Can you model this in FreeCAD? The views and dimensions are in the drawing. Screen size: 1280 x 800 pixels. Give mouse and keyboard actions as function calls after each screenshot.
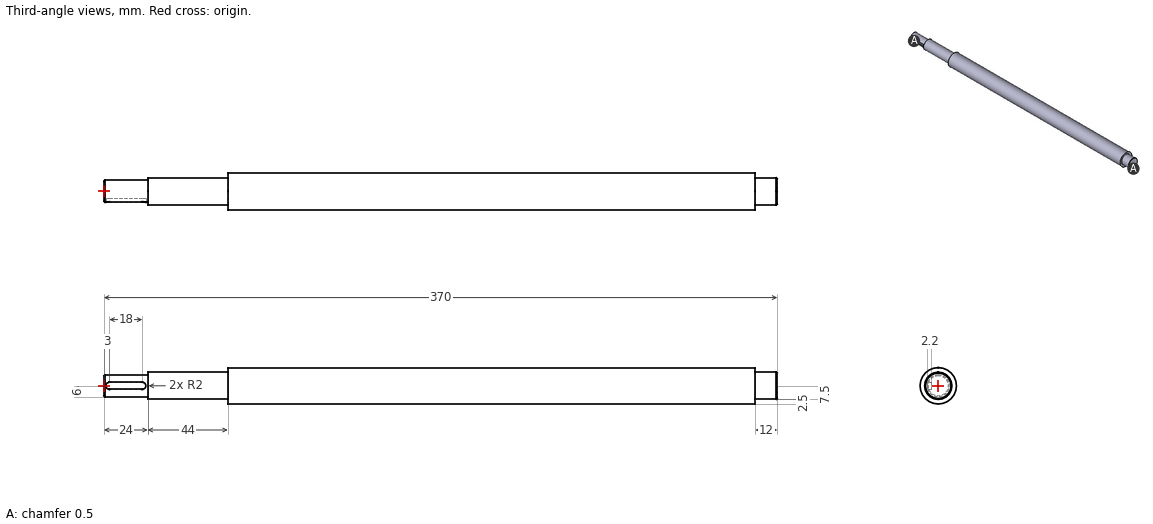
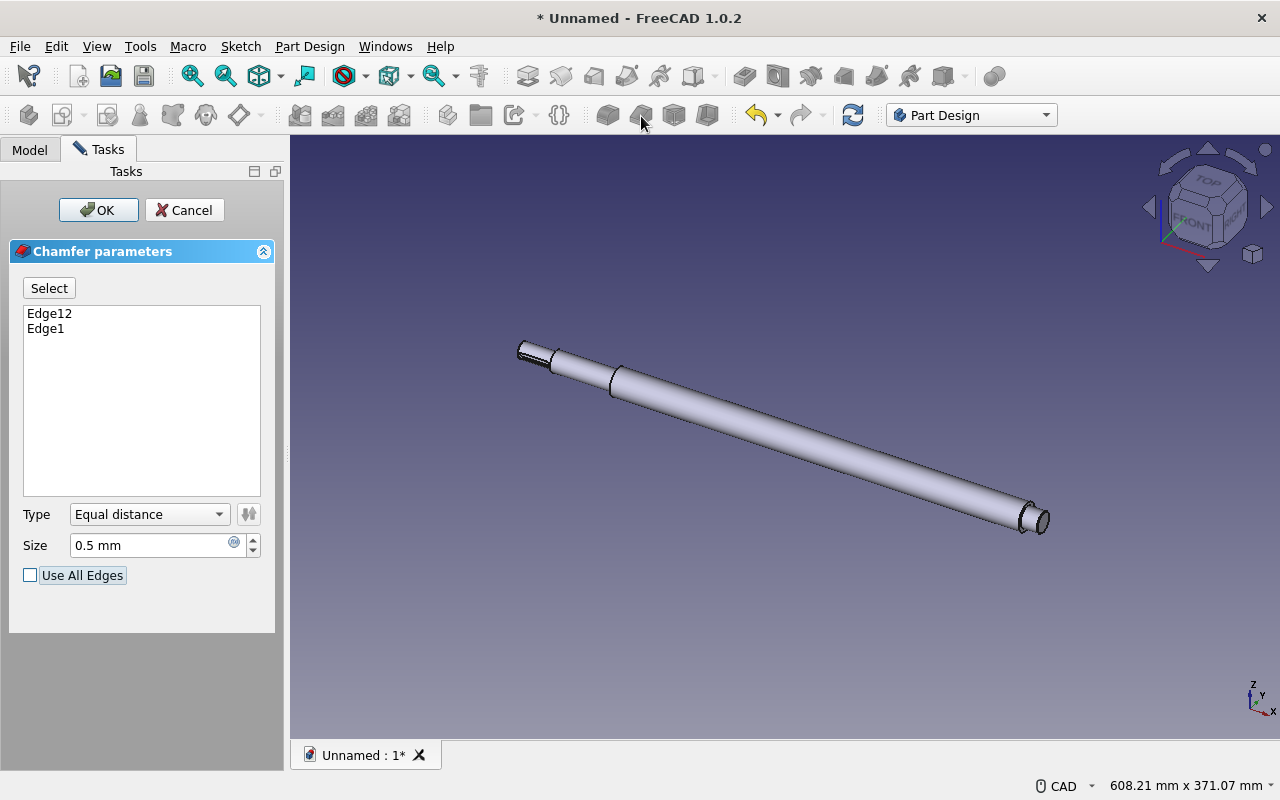
click(99, 210)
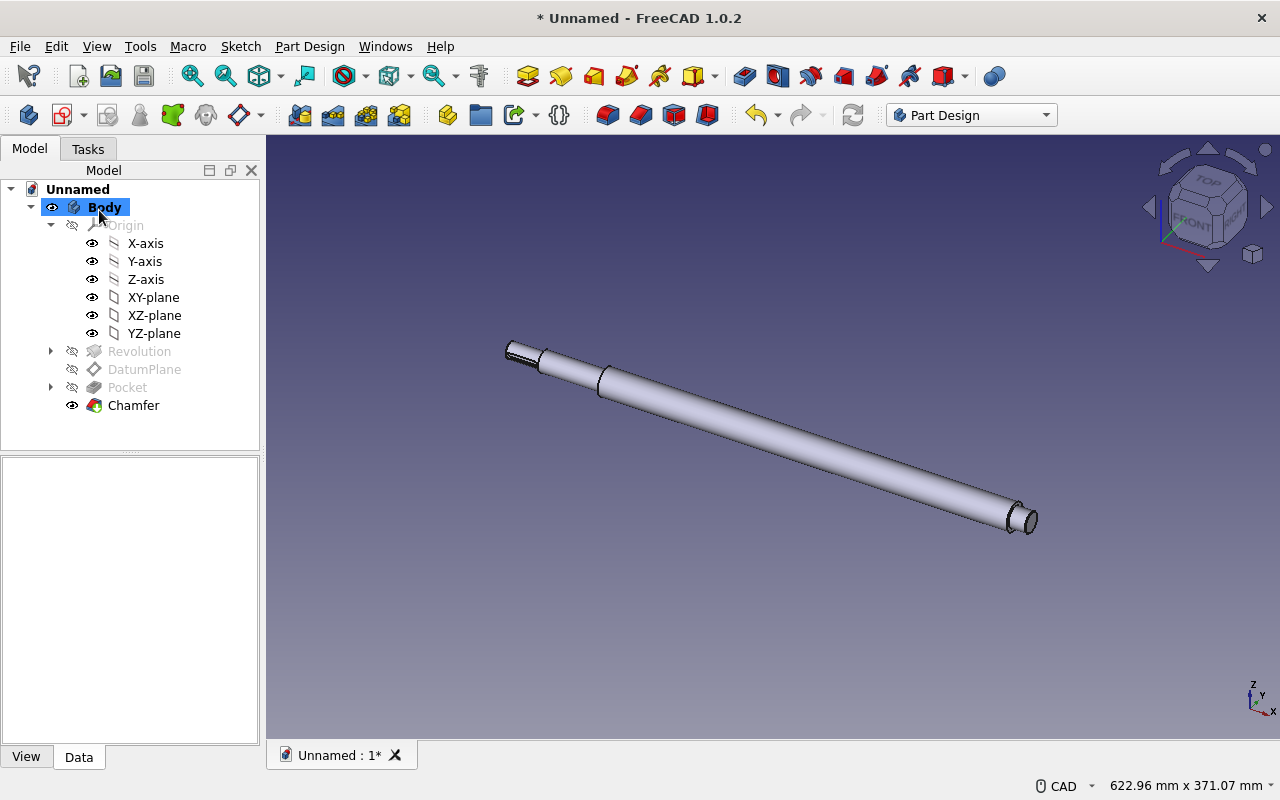
key(0)